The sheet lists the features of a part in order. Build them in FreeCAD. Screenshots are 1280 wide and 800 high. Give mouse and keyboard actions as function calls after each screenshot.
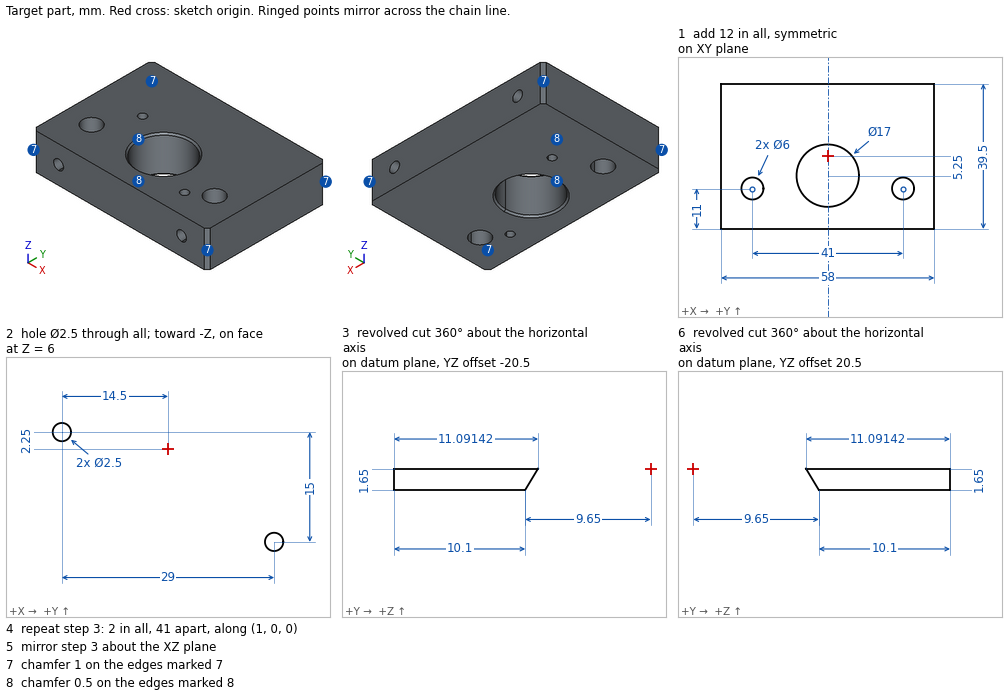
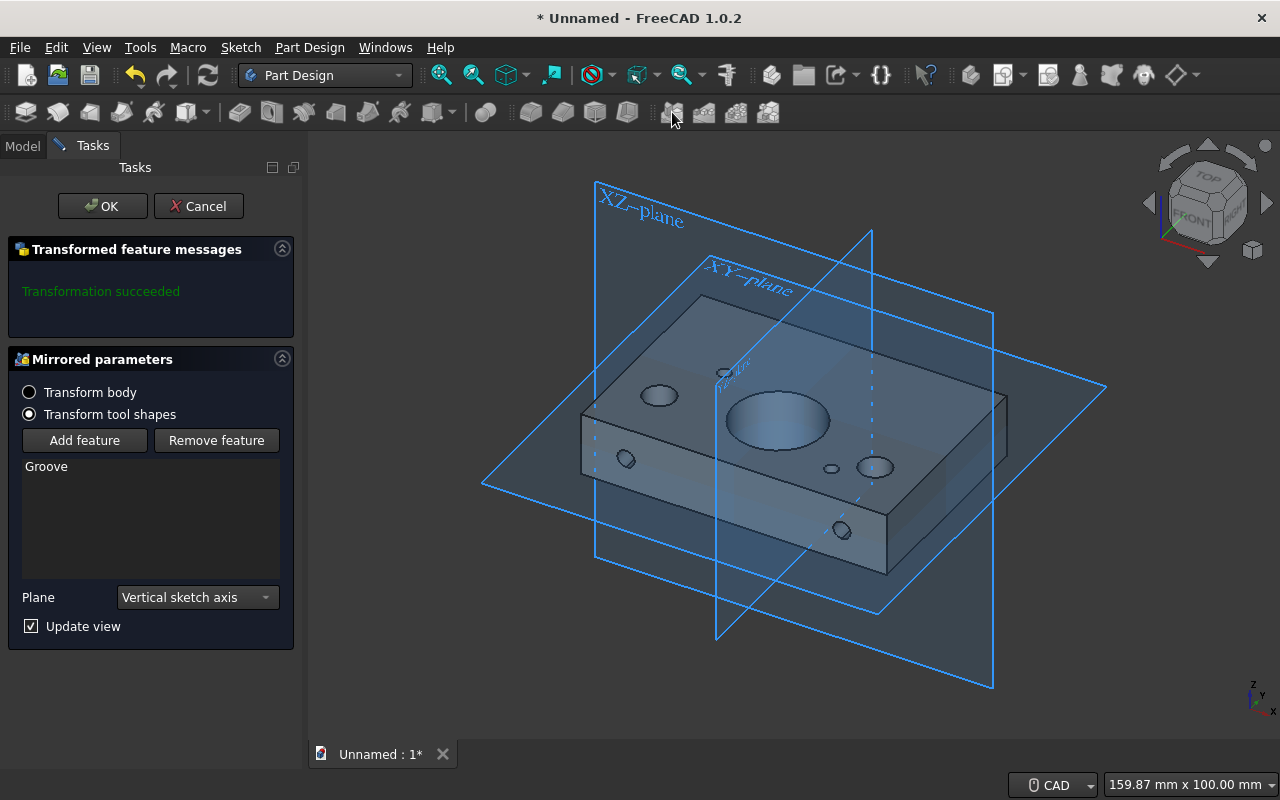
click(198, 598)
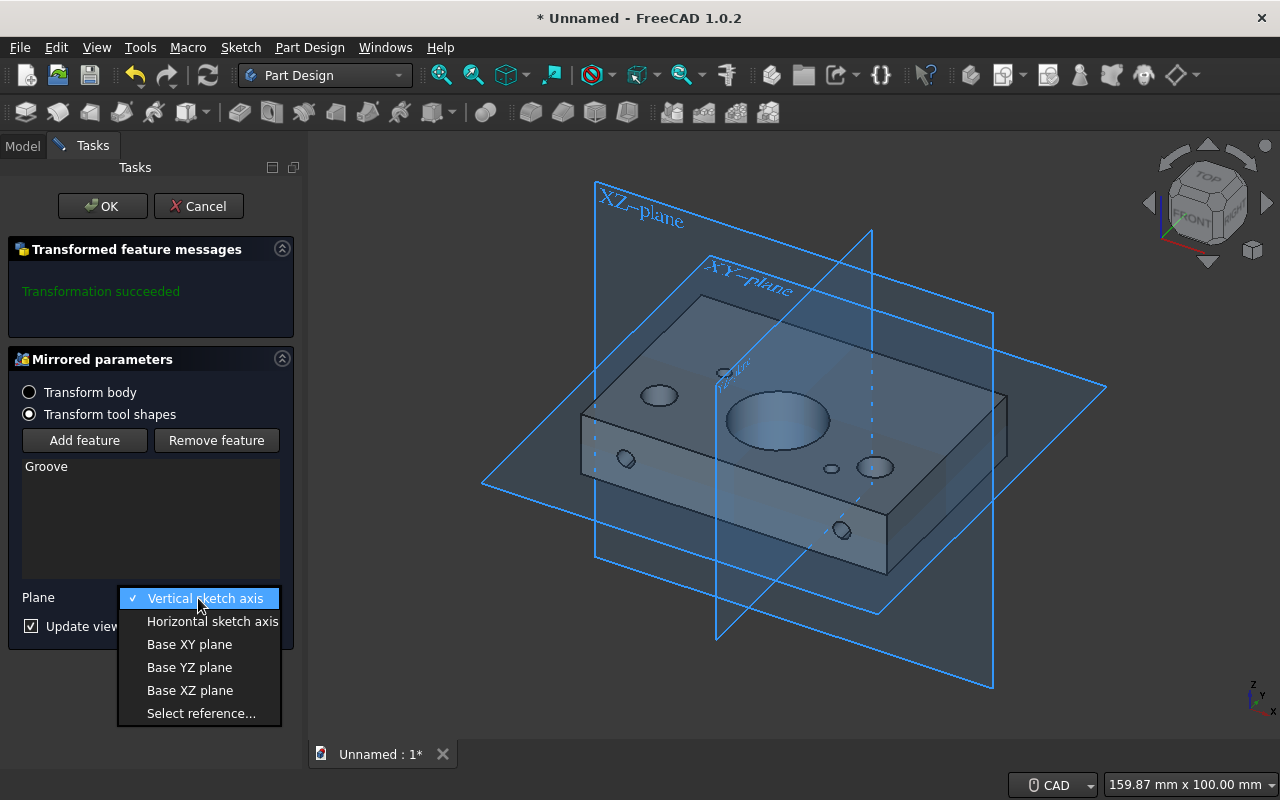
click(198, 690)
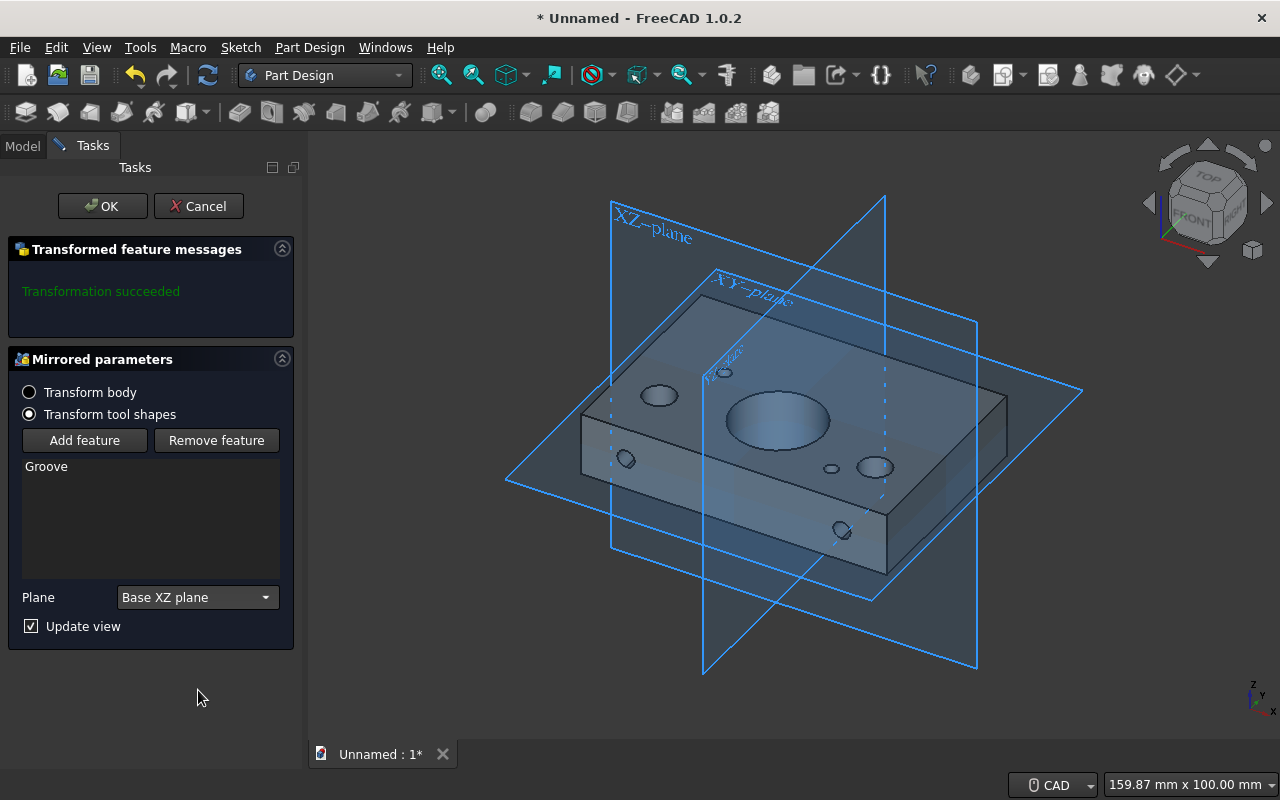
click(103, 206)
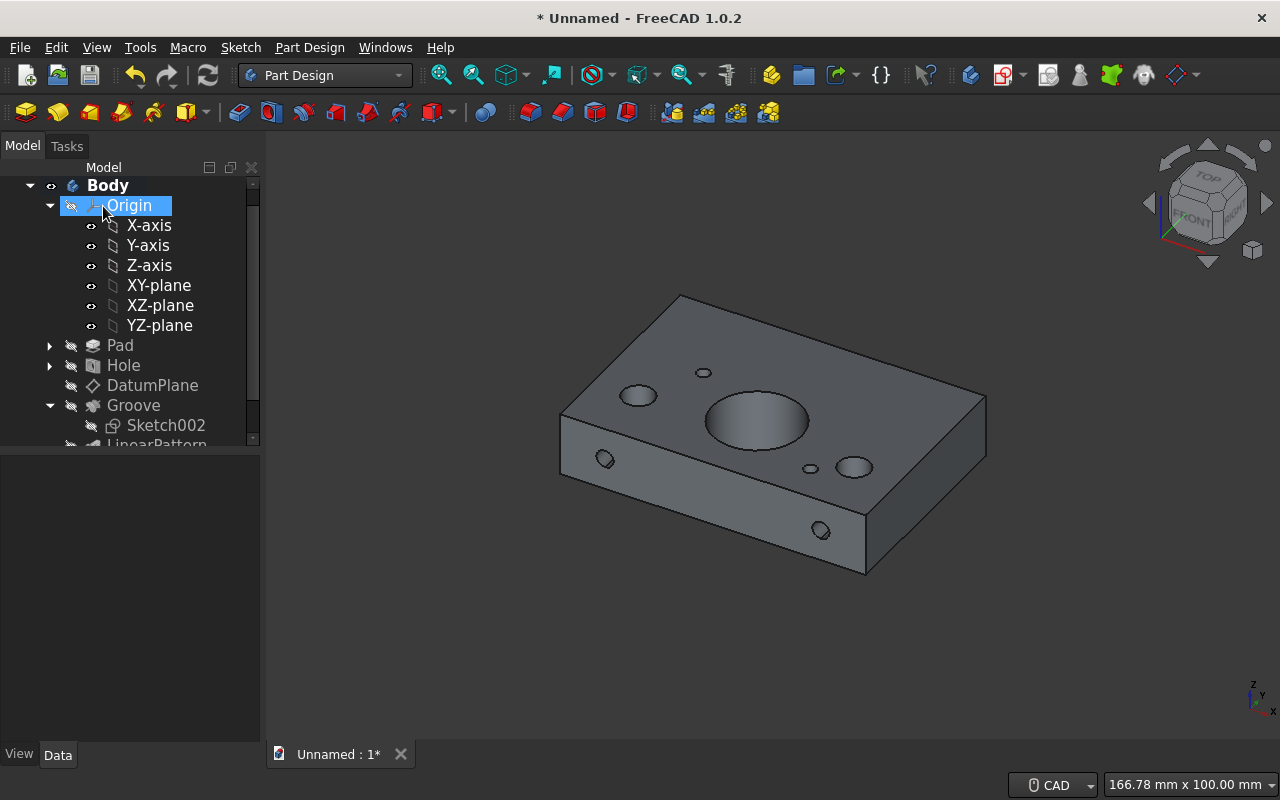
click(136, 326)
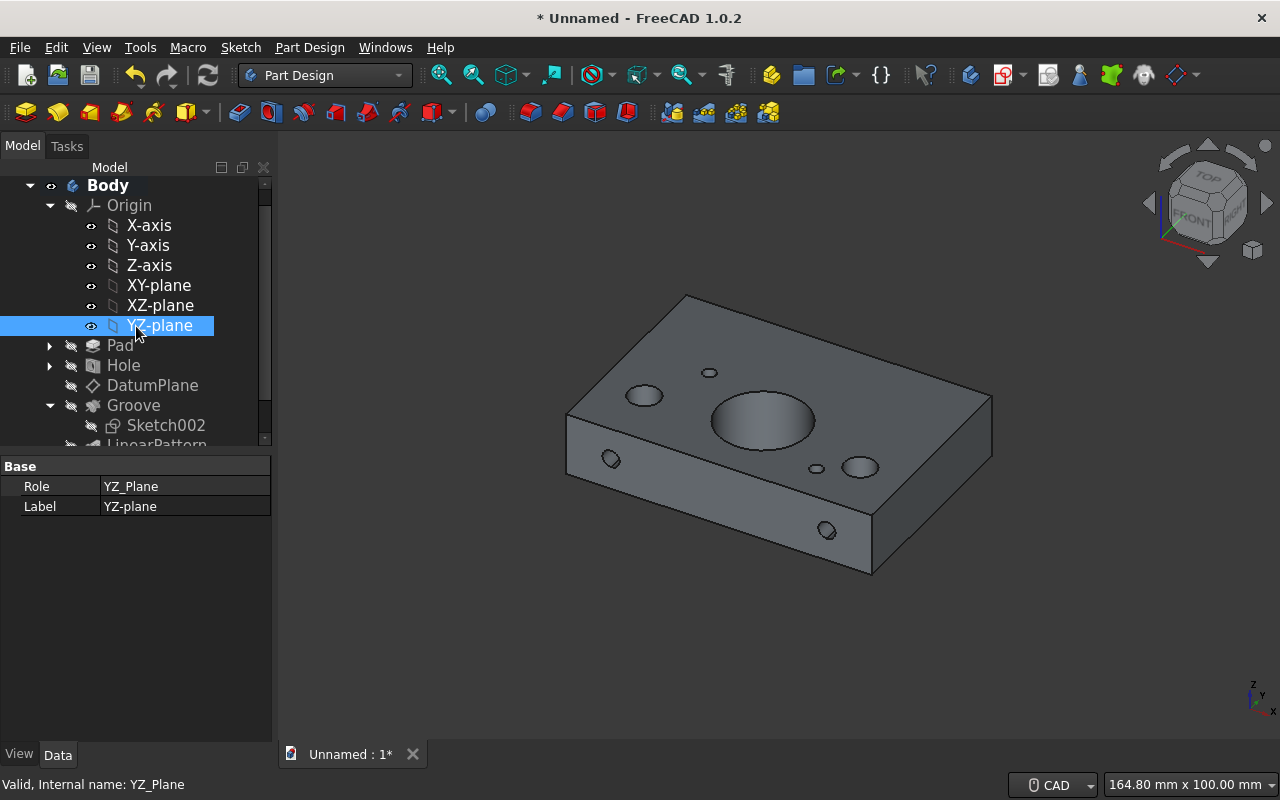
click(1176, 76)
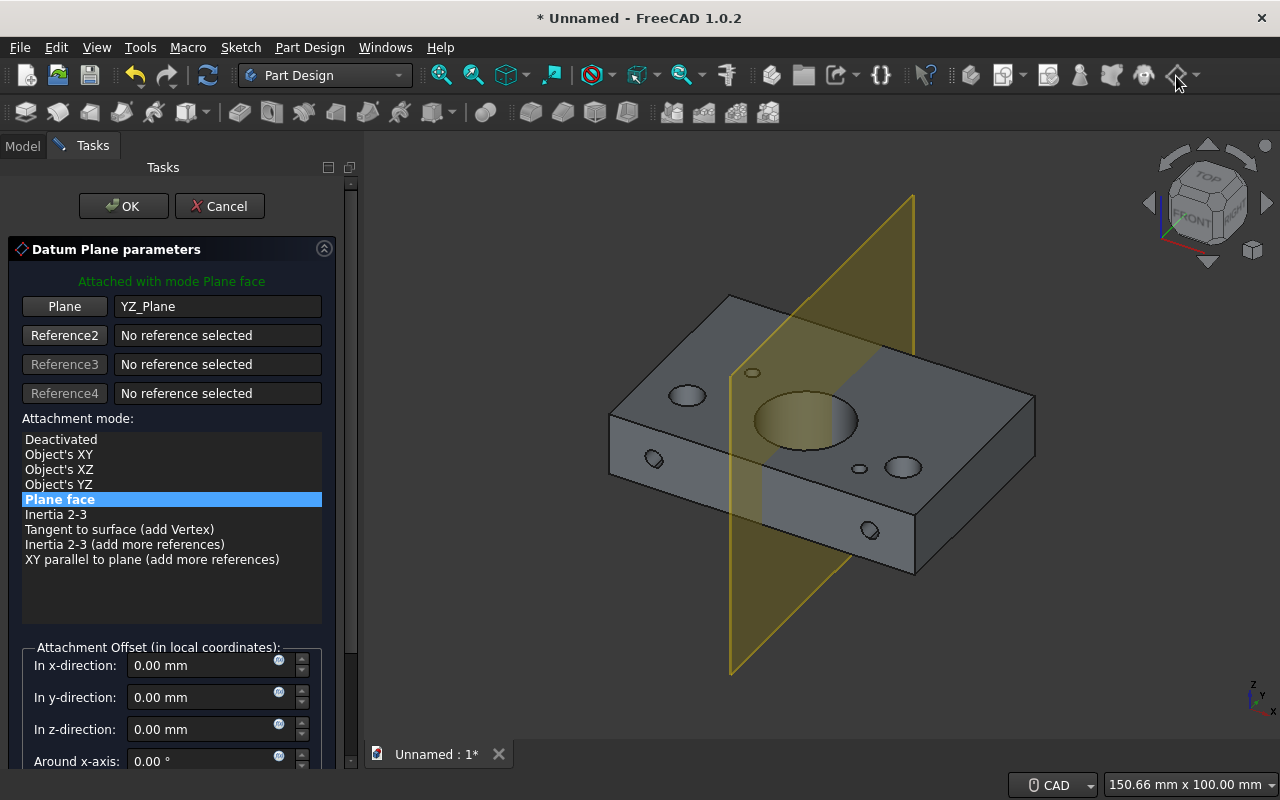
triple_click(210, 729)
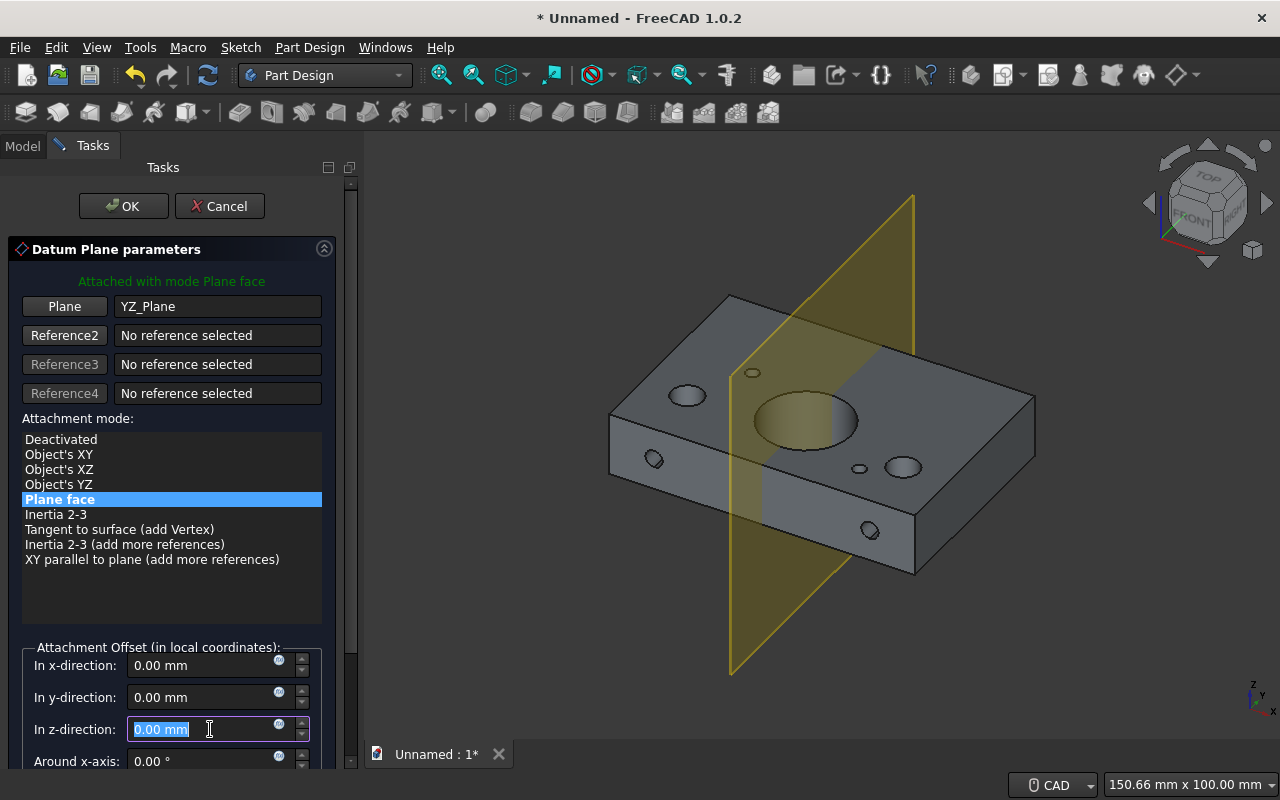
text(20.5)
key(Tab)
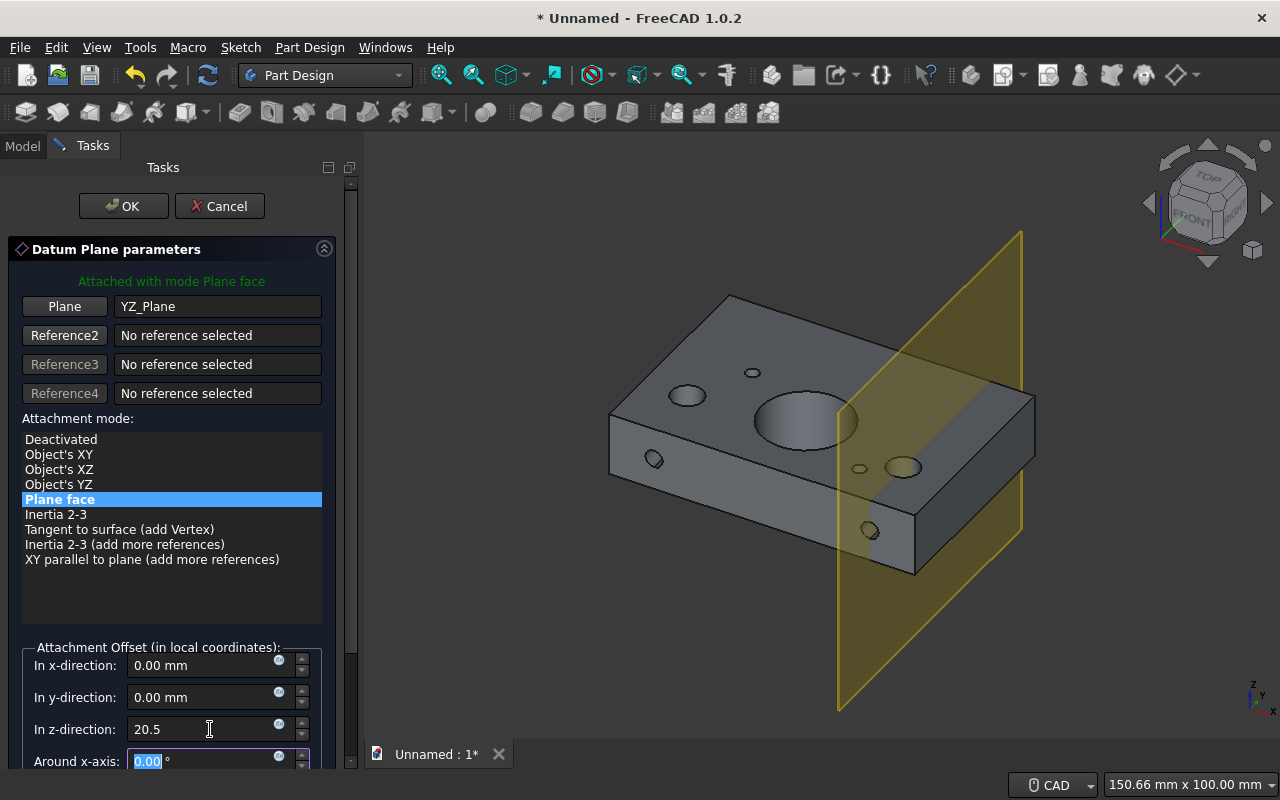
click(124, 206)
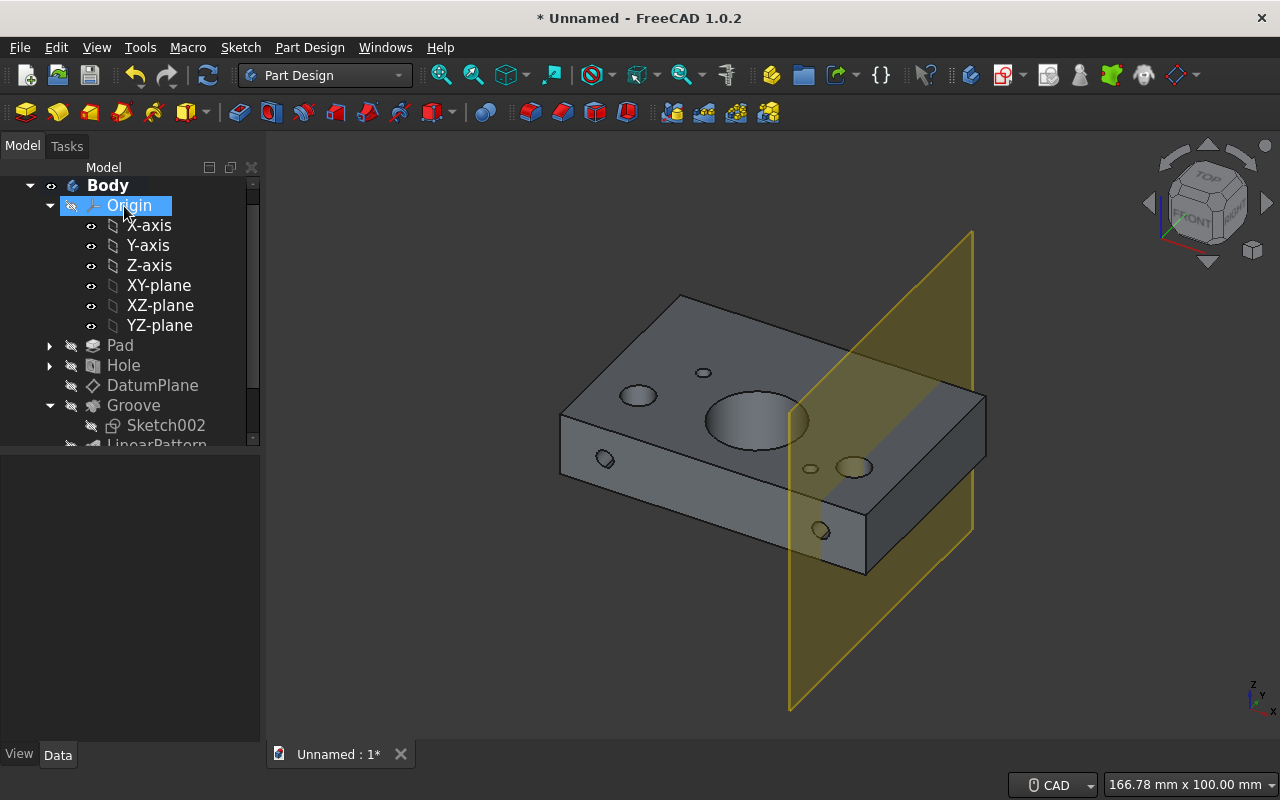
scroll(120, 321, down, 3)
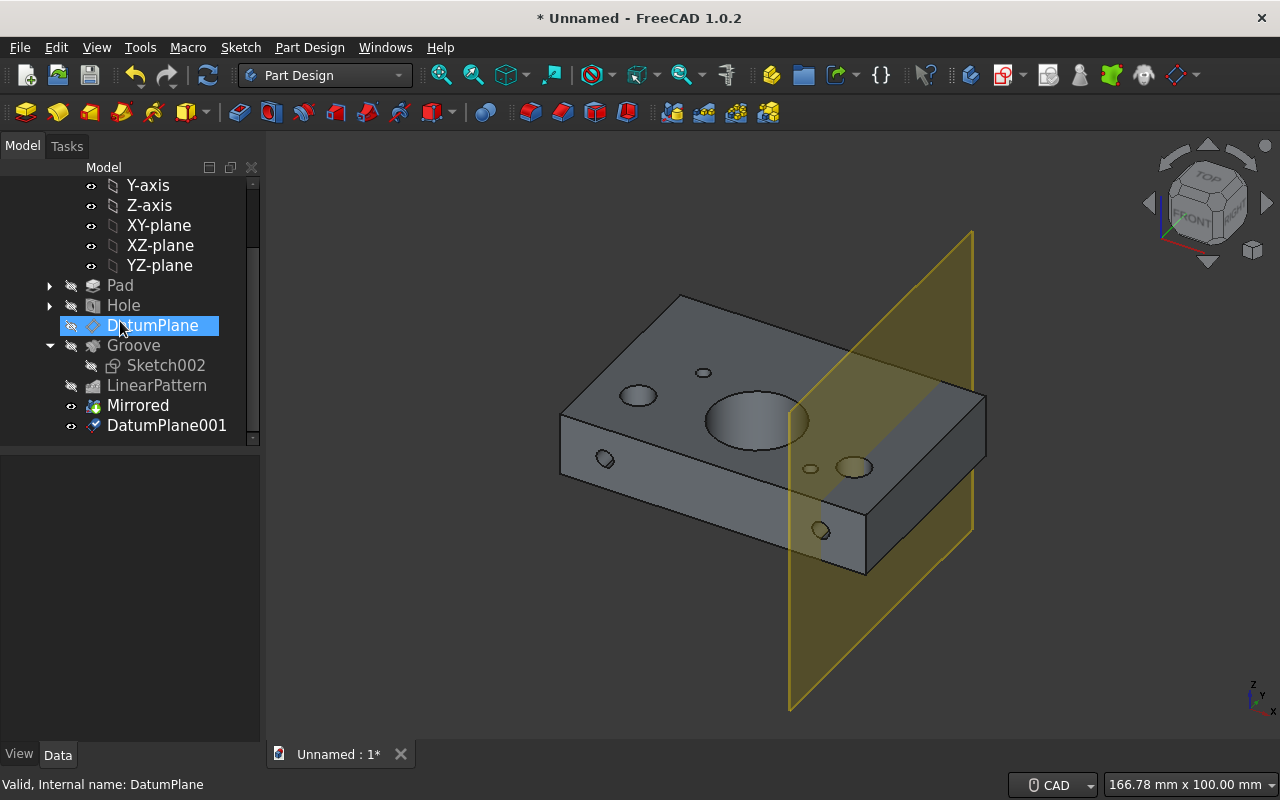
click(116, 426)